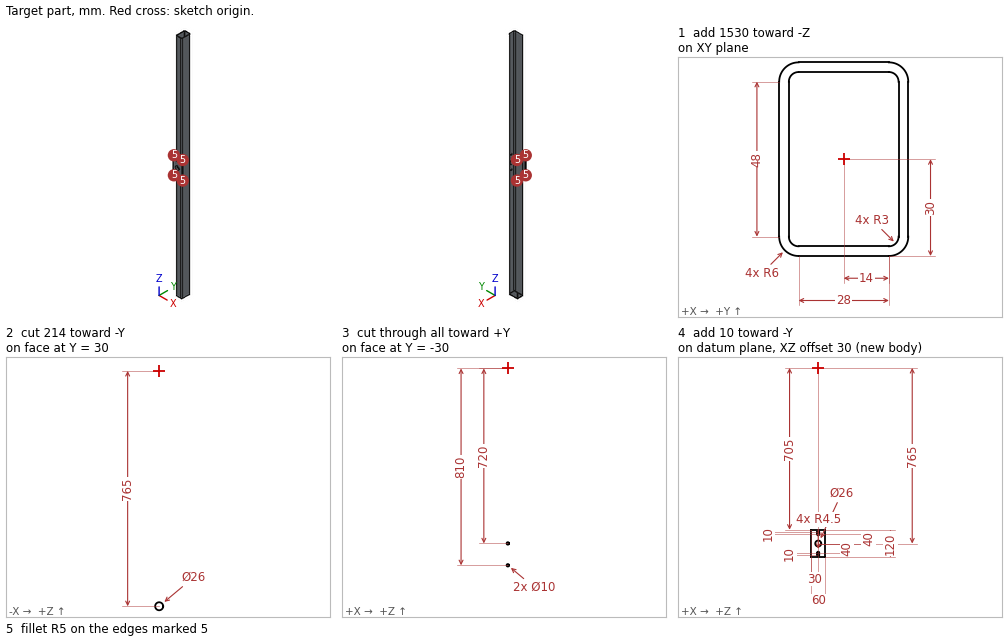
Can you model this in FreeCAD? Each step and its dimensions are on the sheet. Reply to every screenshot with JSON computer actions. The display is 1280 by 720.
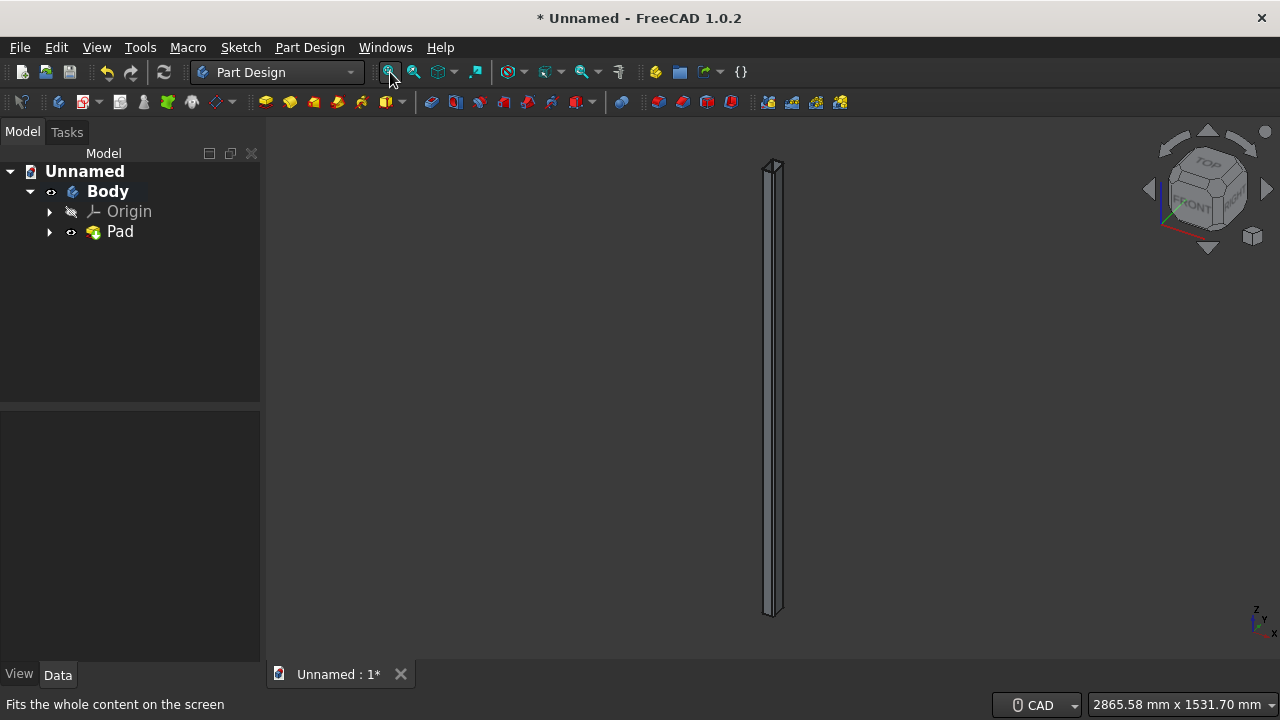
{"action": "key", "text": "4"}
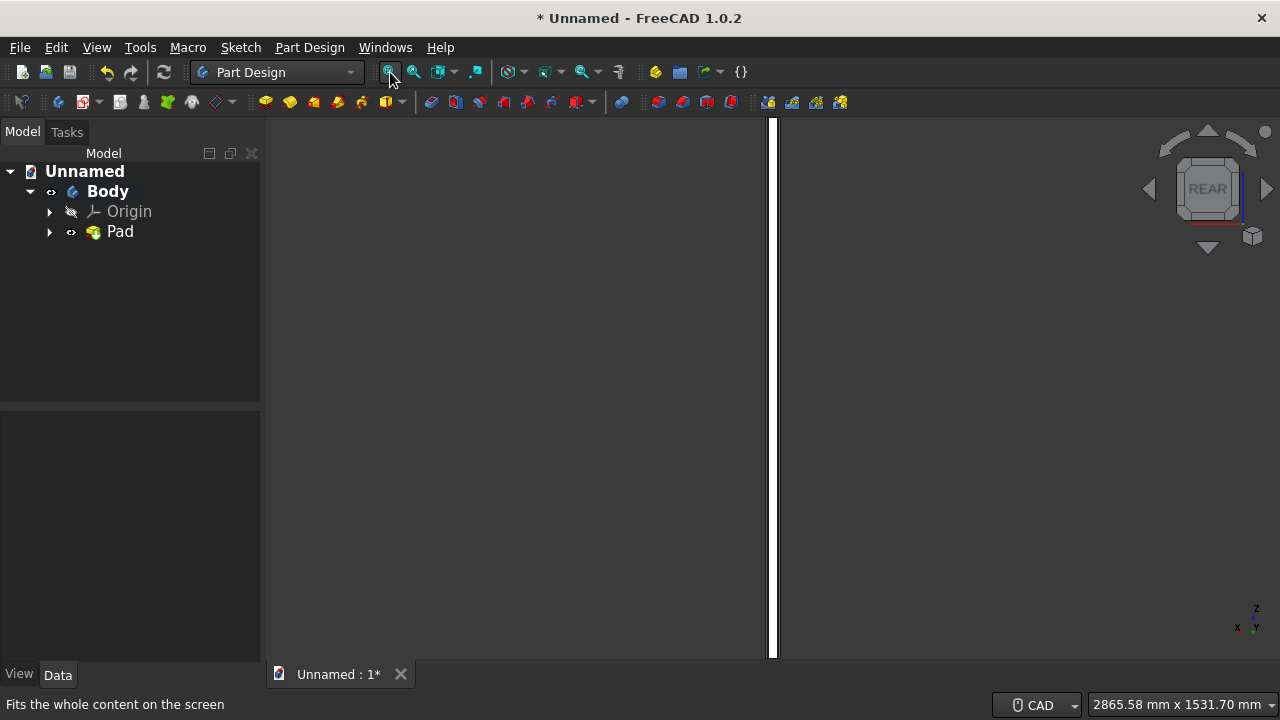
{"action": "left_click", "coordinate": [390, 72]}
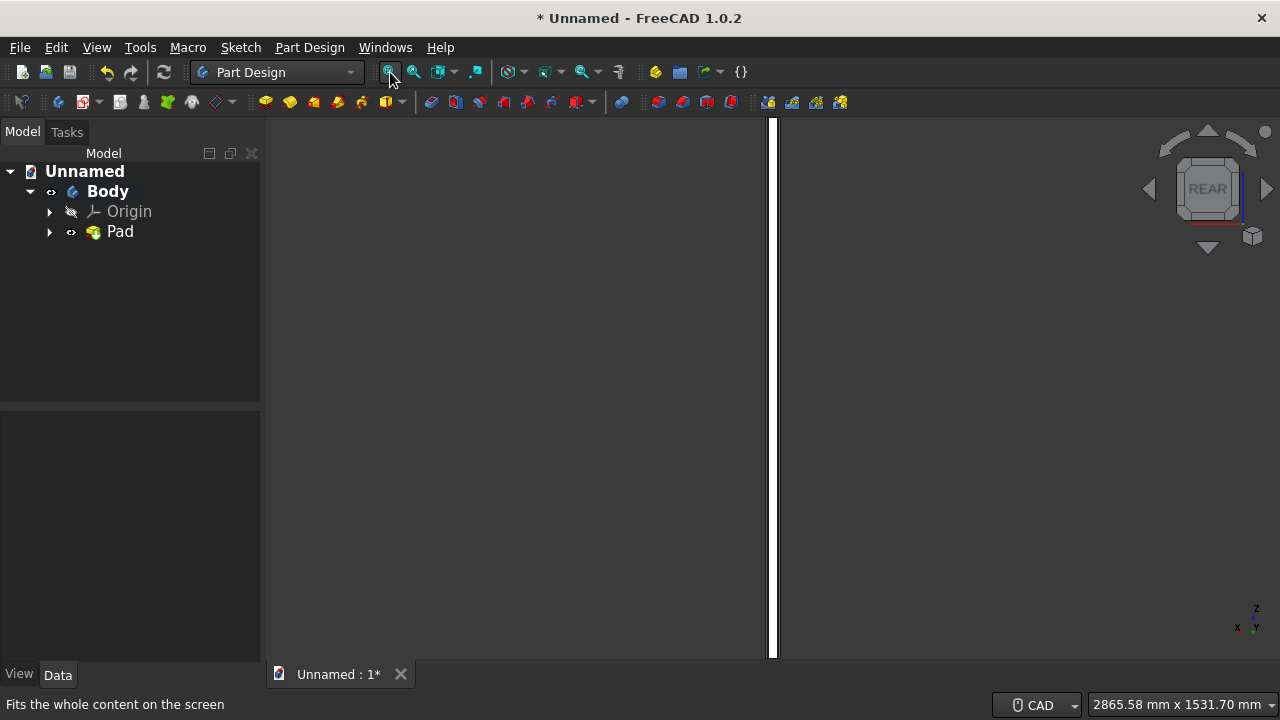
{"action": "scroll", "coordinate": [773, 155], "scroll_direction": "up", "scroll_amount": 5}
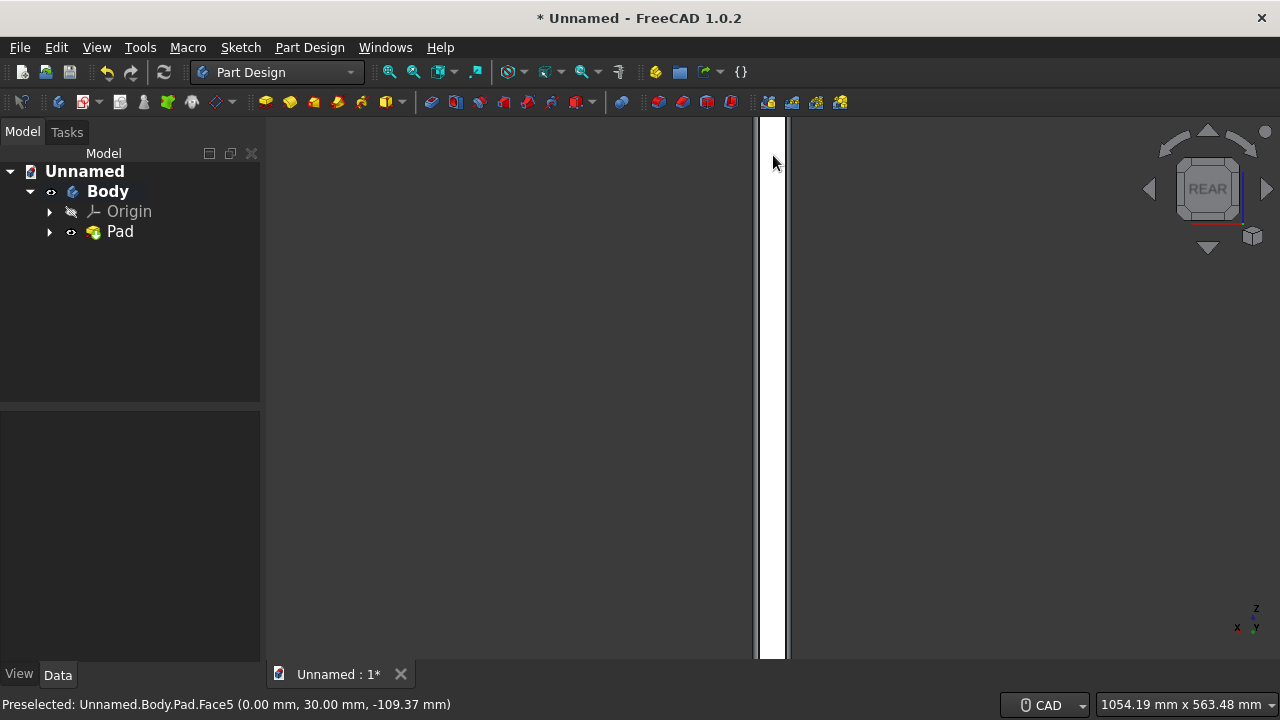
{"action": "left_click", "coordinate": [772, 157]}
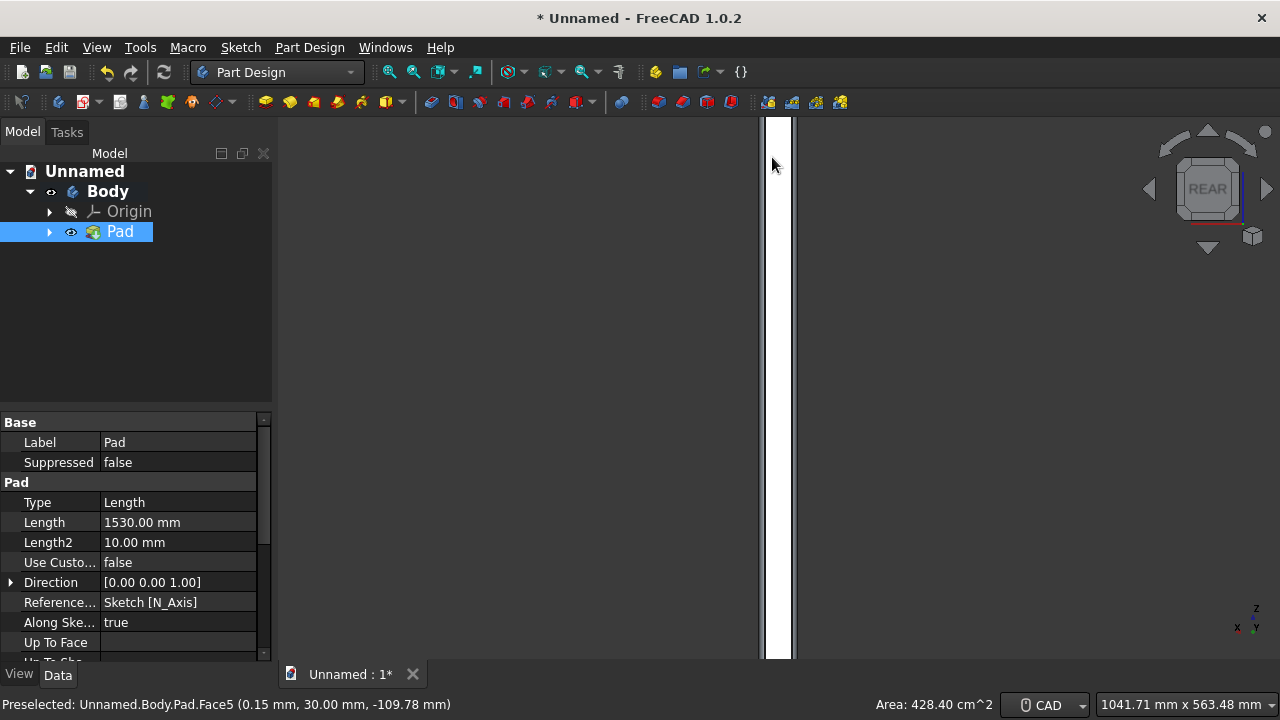
{"action": "left_click", "coordinate": [84, 102]}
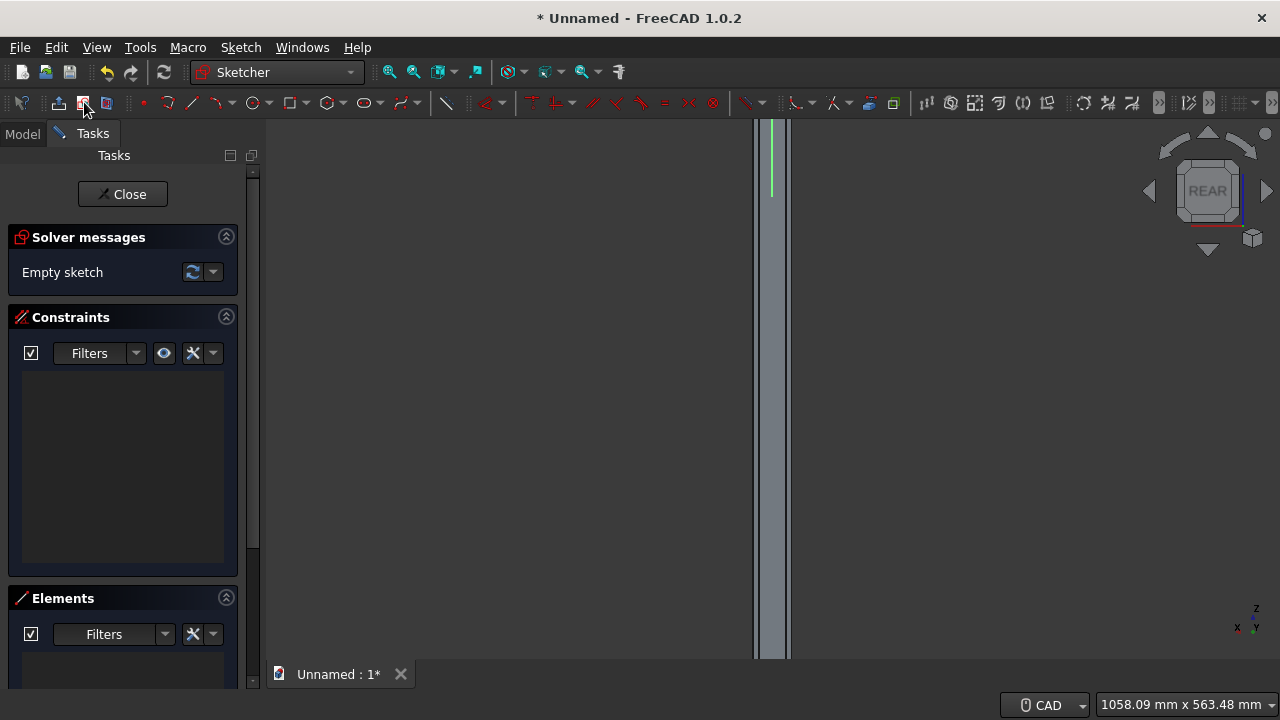
{"action": "scroll", "coordinate": [704, 389], "scroll_direction": "down", "scroll_amount": 5}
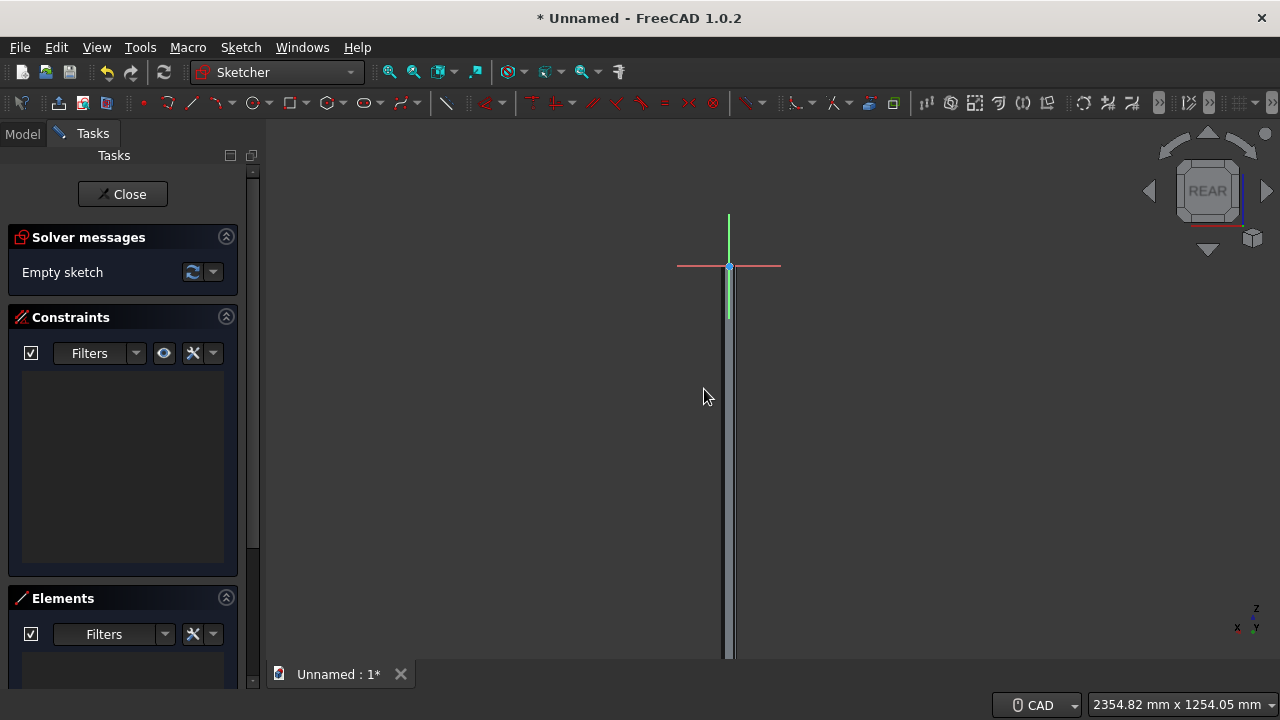
{"action": "scroll", "coordinate": [731, 544], "scroll_direction": "up", "scroll_amount": 15}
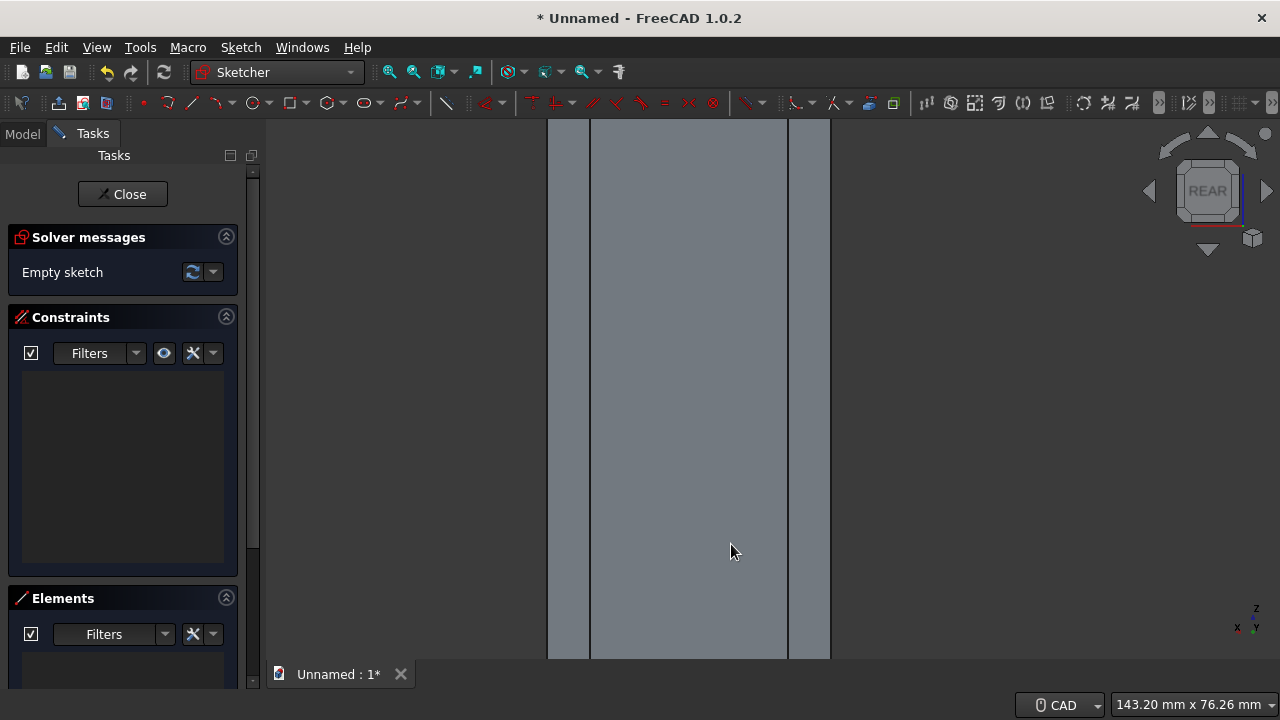
{"action": "scroll", "coordinate": [670, 344], "scroll_direction": "up", "scroll_amount": 3}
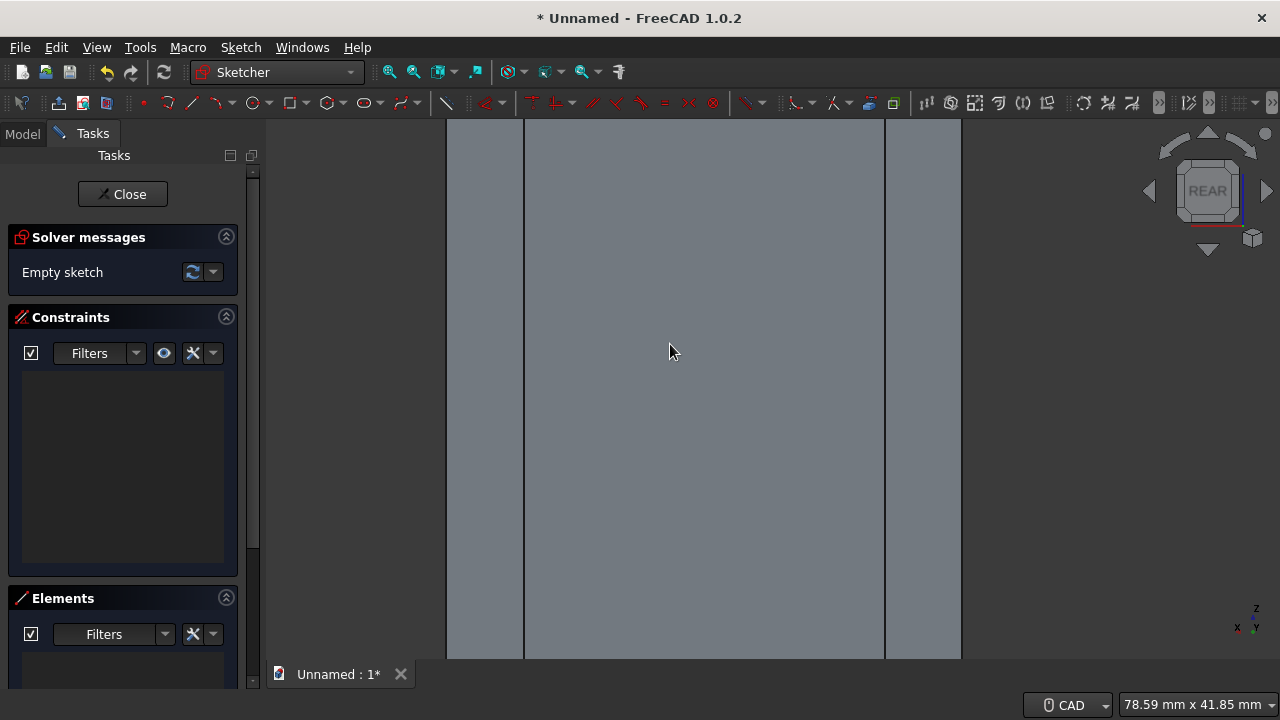
{"action": "left_click", "coordinate": [254, 104]}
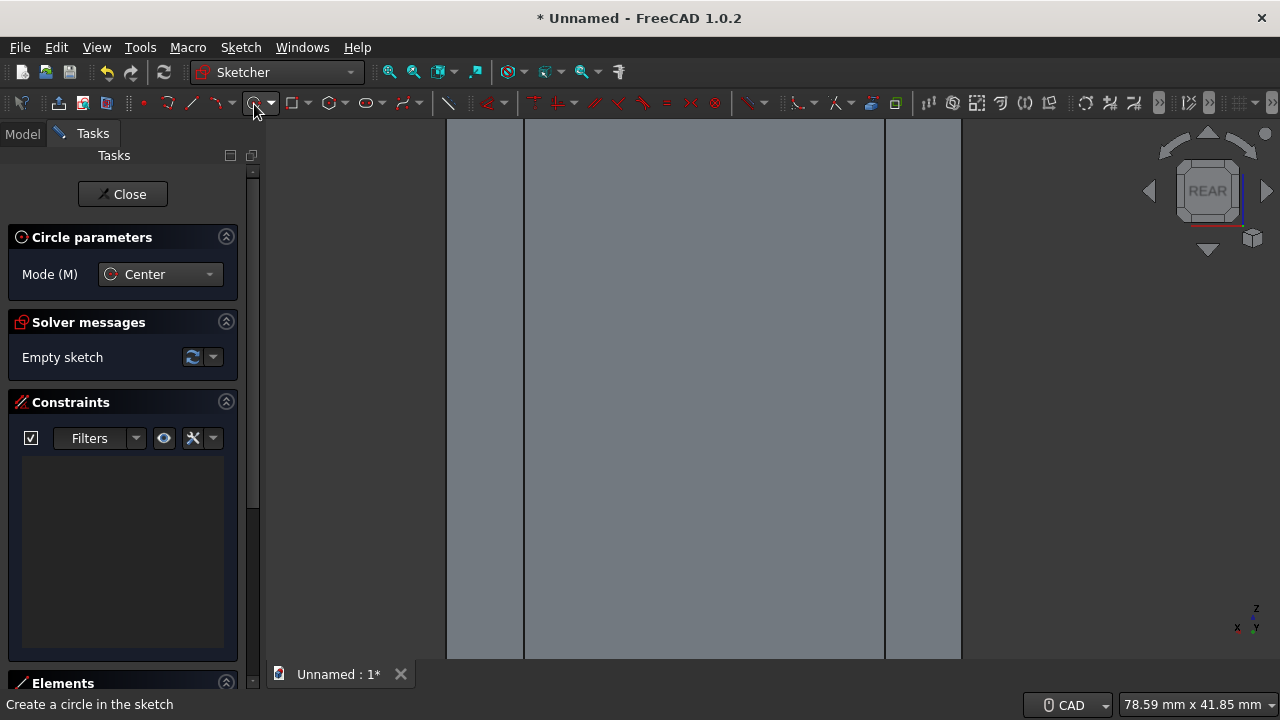
{"action": "left_click", "coordinate": [704, 388]}
{"action": "mouse_move", "coordinate": [823, 270]}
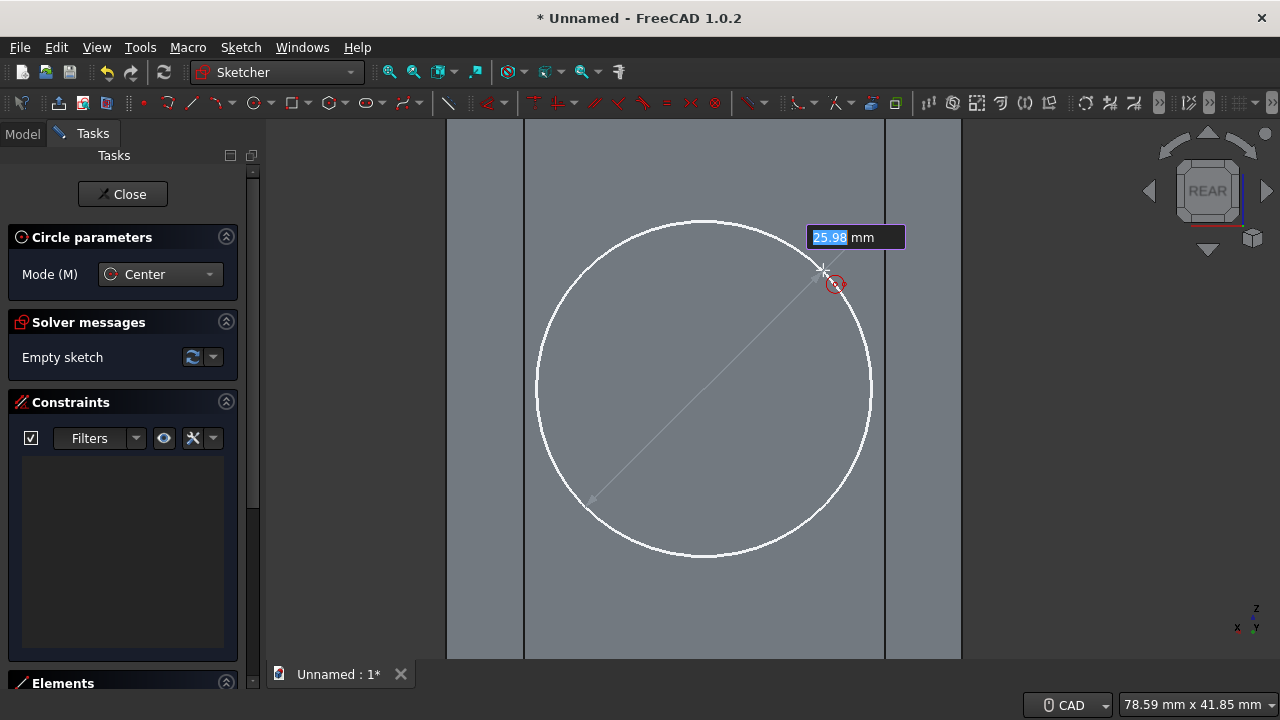
{"action": "type", "text": "26"}
{"action": "key", "text": "Return"}
{"action": "key", "text": "Escape"}